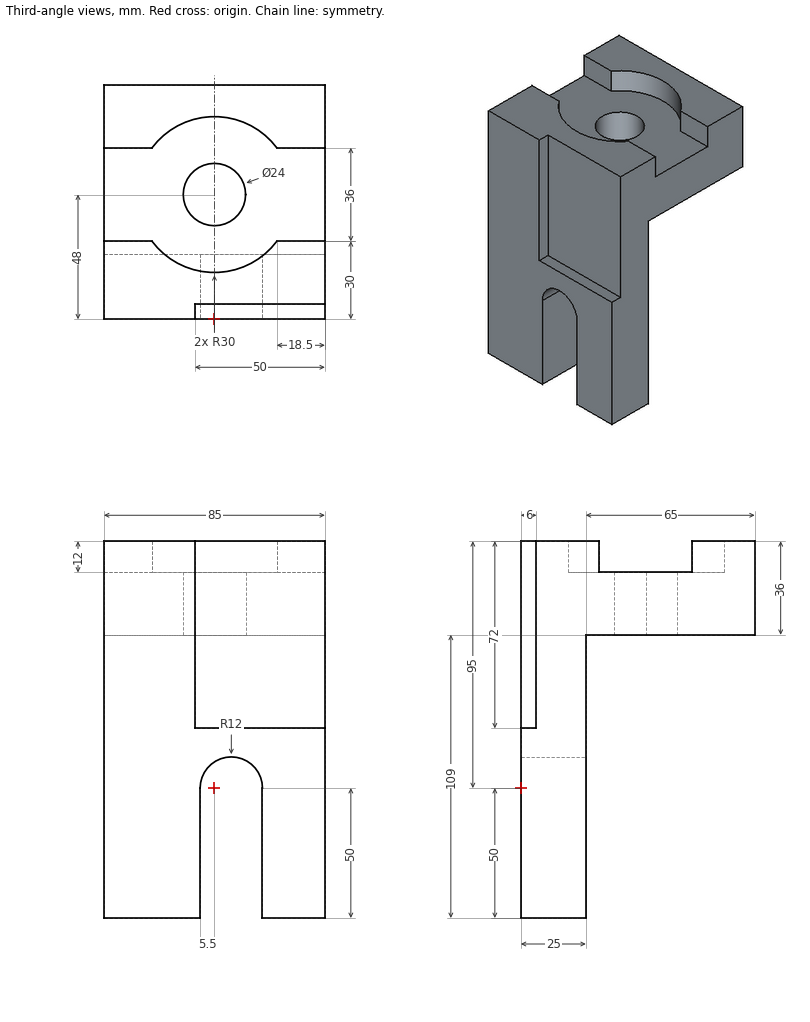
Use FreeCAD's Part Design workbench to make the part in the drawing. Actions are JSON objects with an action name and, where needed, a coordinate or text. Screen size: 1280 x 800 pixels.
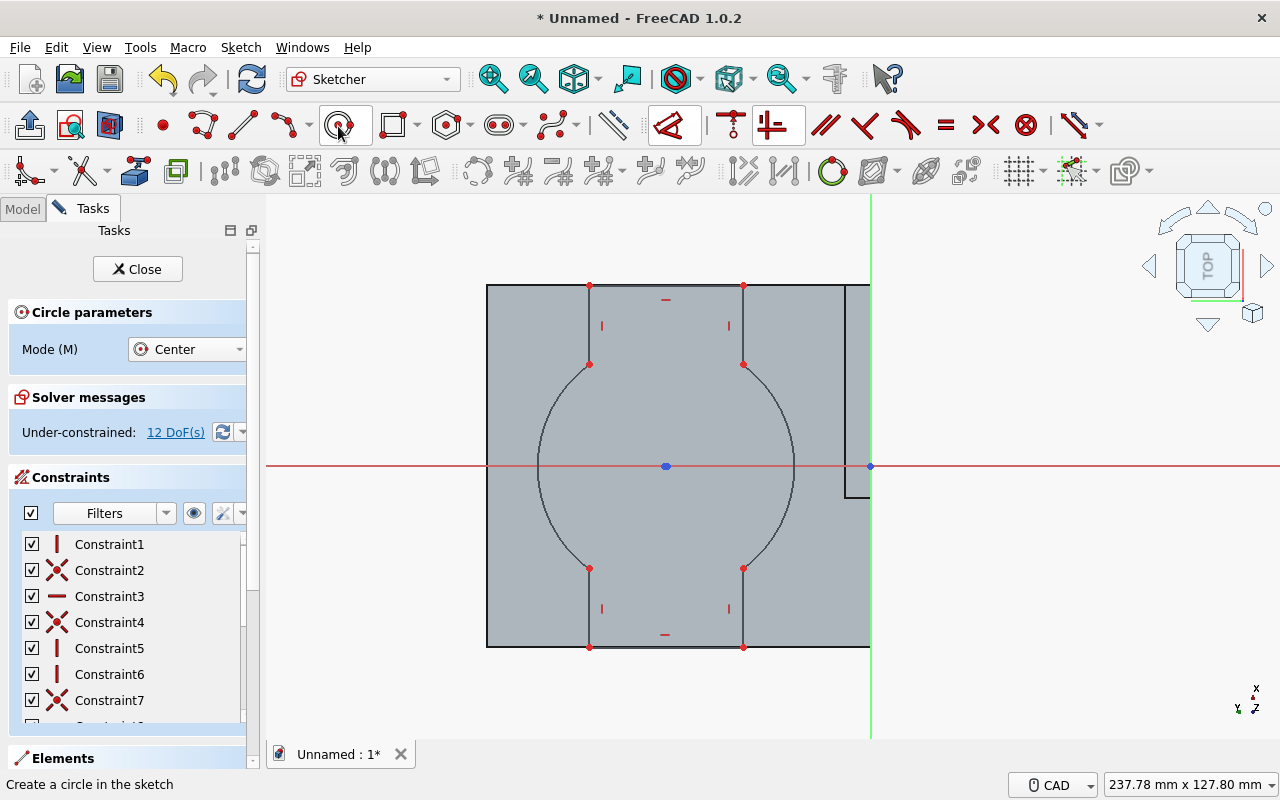
{"action": "left_click", "coordinate": [666, 466]}
{"action": "left_click", "coordinate": [702, 430]}
{"action": "key", "text": "Escape"}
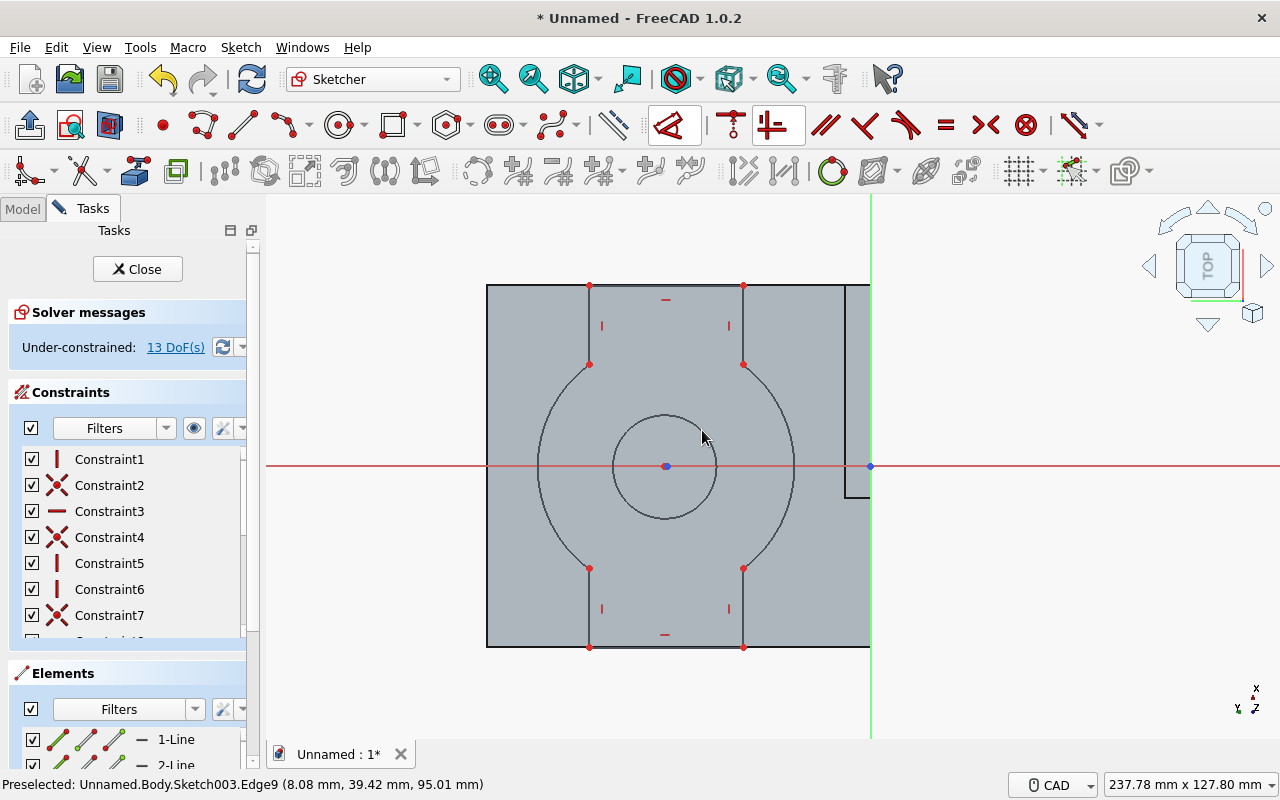
{"action": "left_click", "coordinate": [701, 430]}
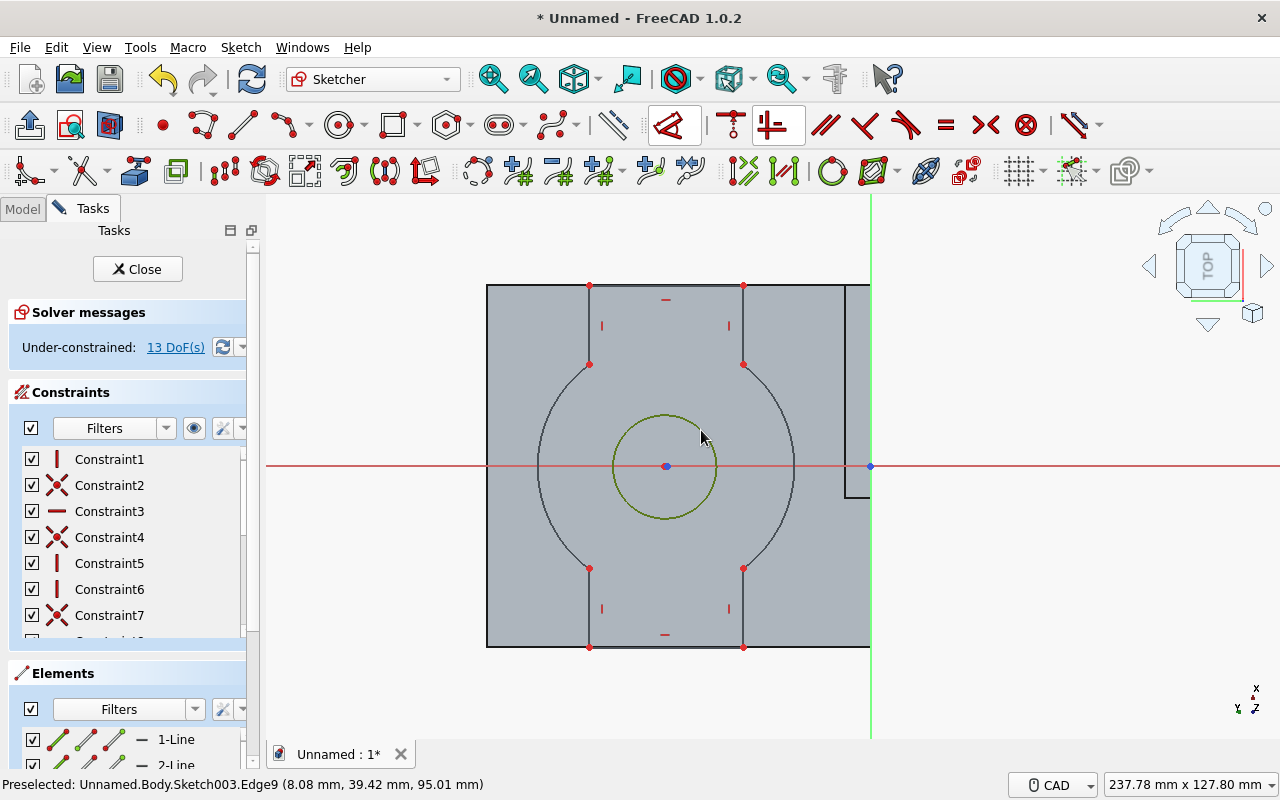
{"action": "left_click", "coordinate": [786, 513]}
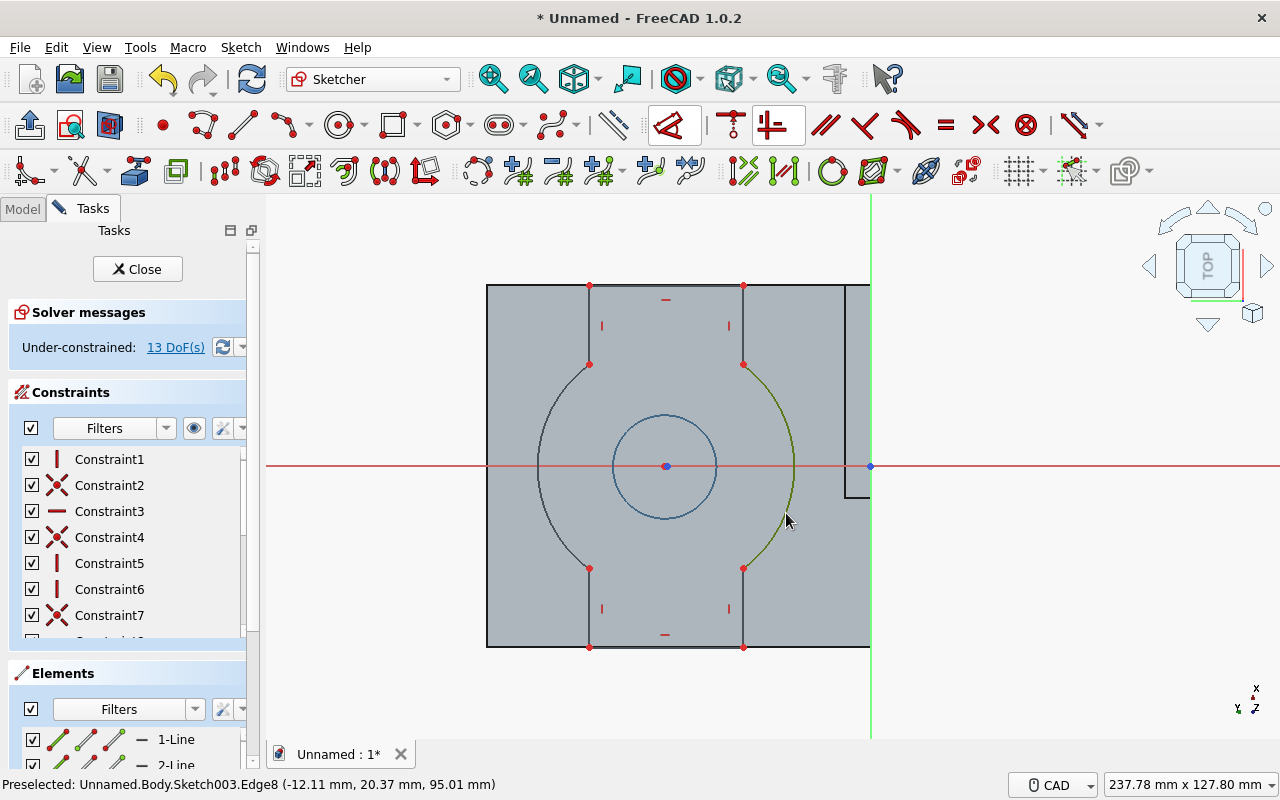
{"action": "left_click", "coordinate": [732, 126]}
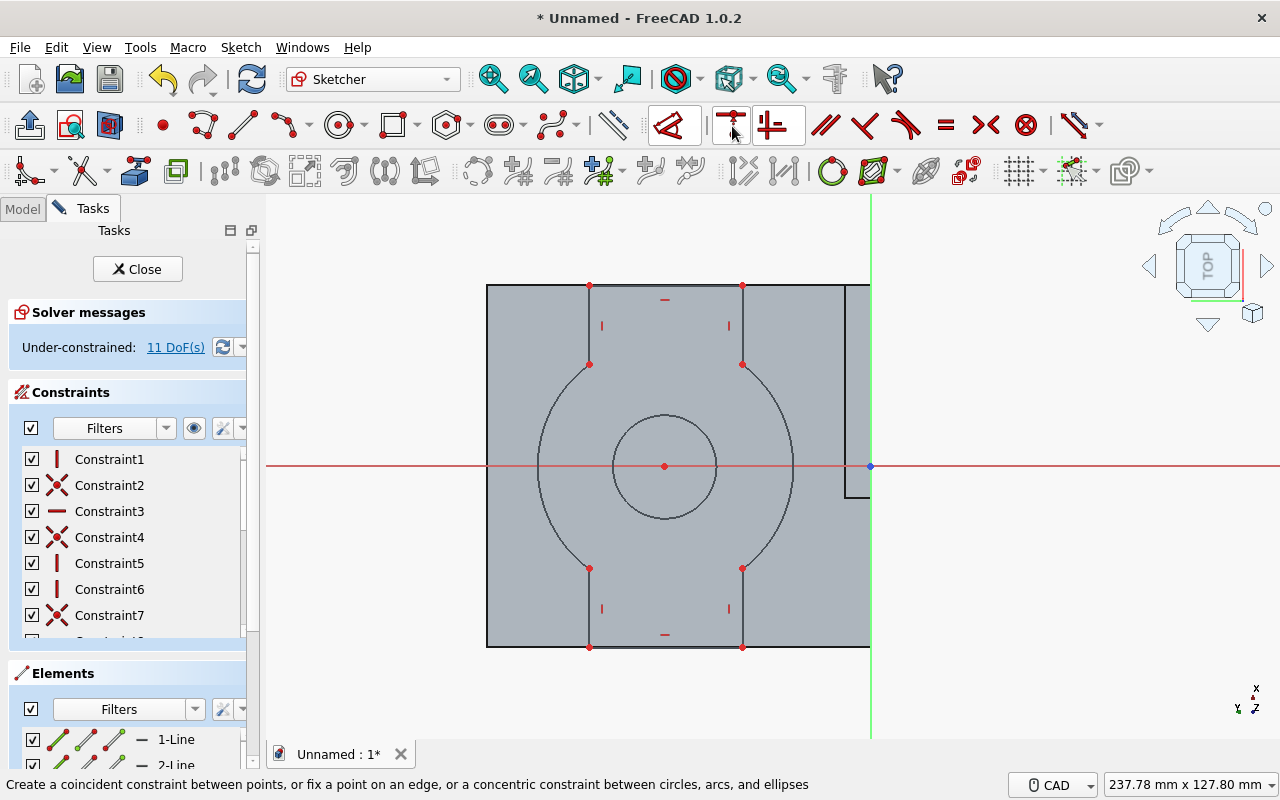
{"action": "left_click", "coordinate": [546, 421]}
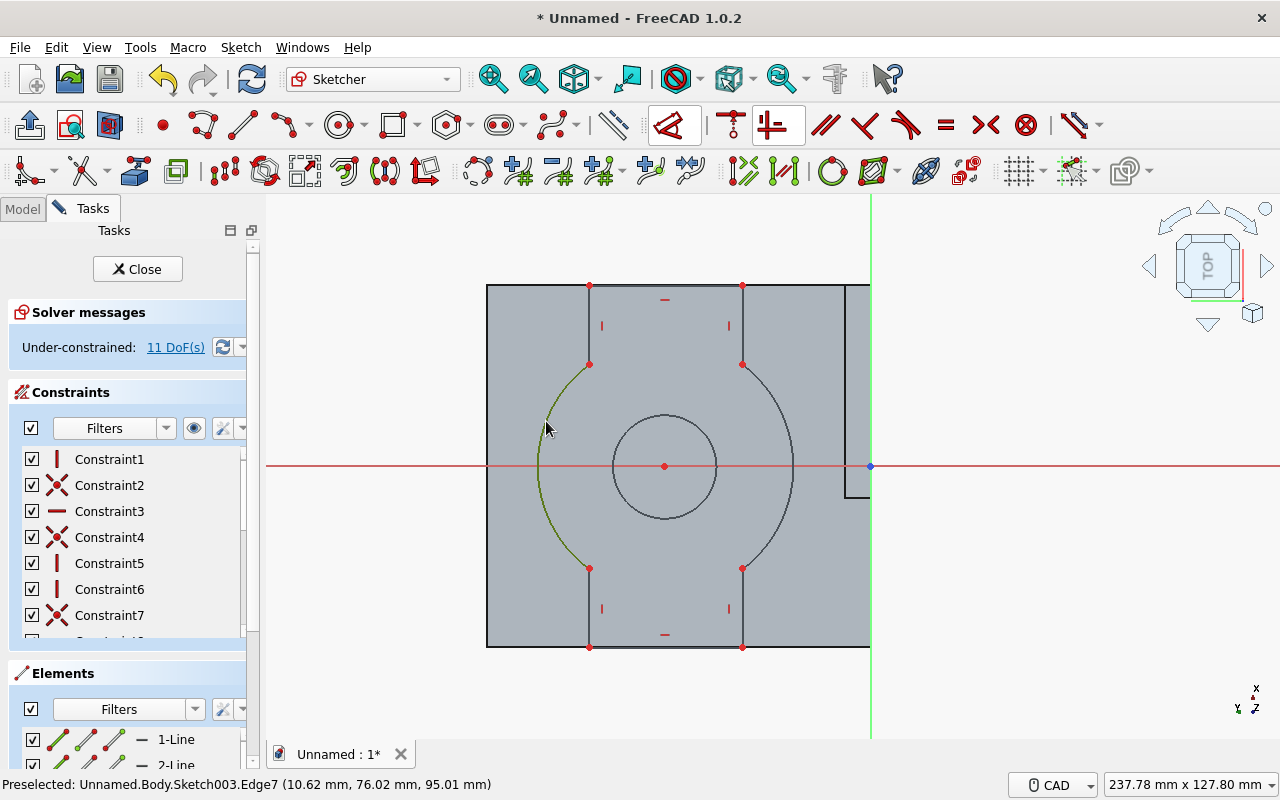
{"action": "left_click", "coordinate": [785, 513]}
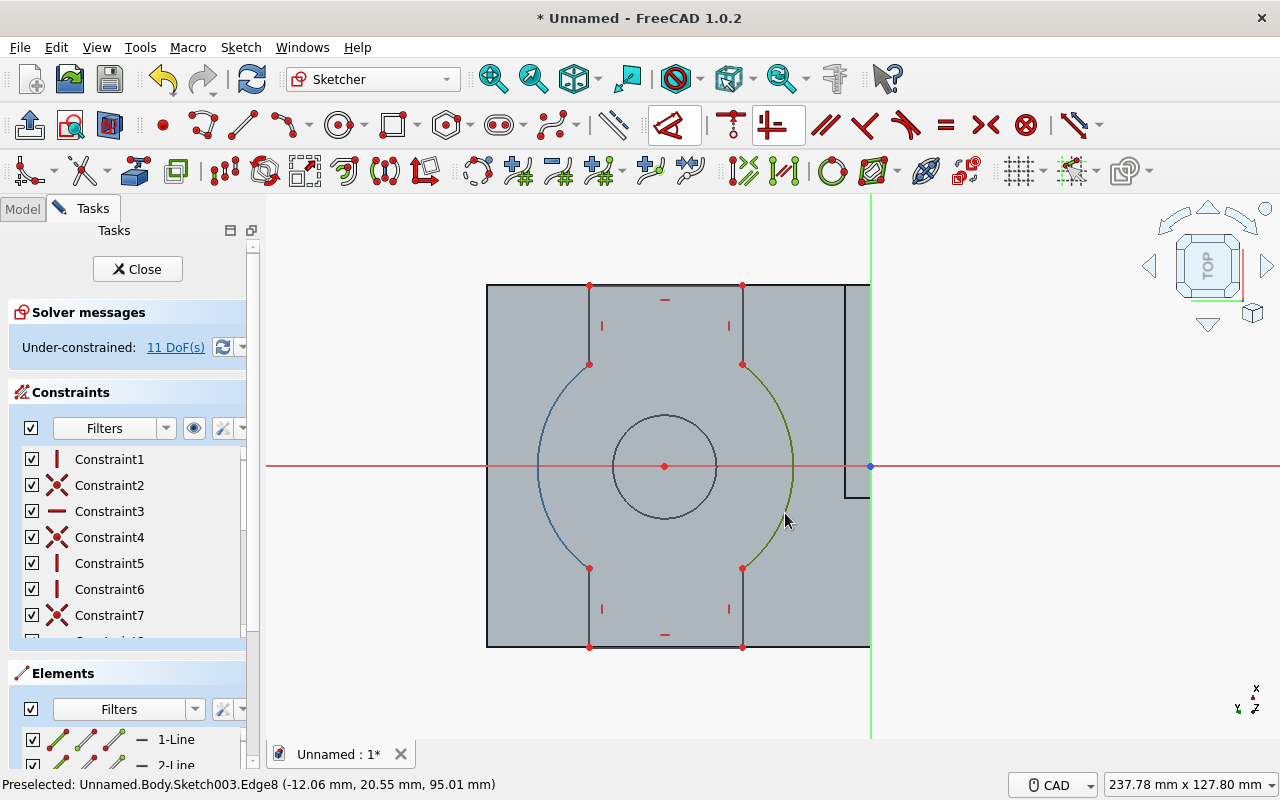
{"action": "left_click", "coordinate": [946, 126]}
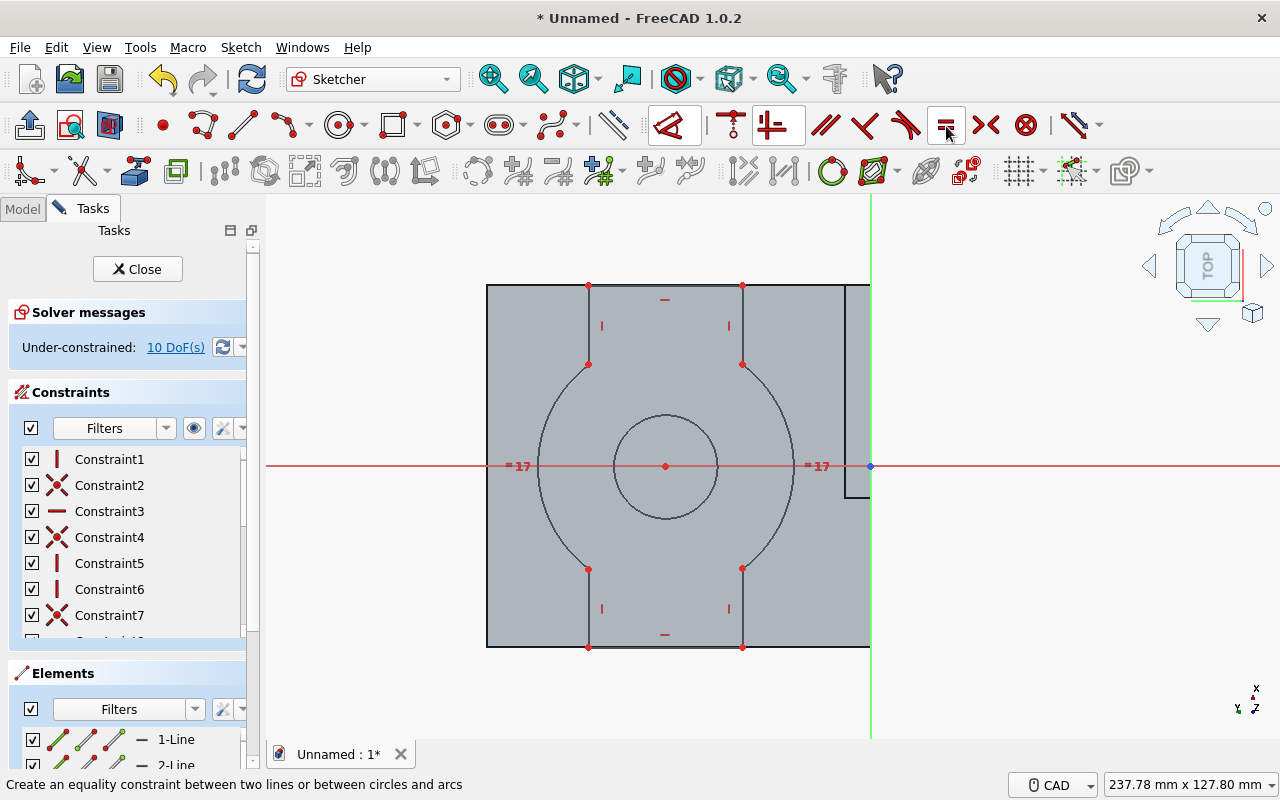
{"action": "left_click", "coordinate": [666, 467]}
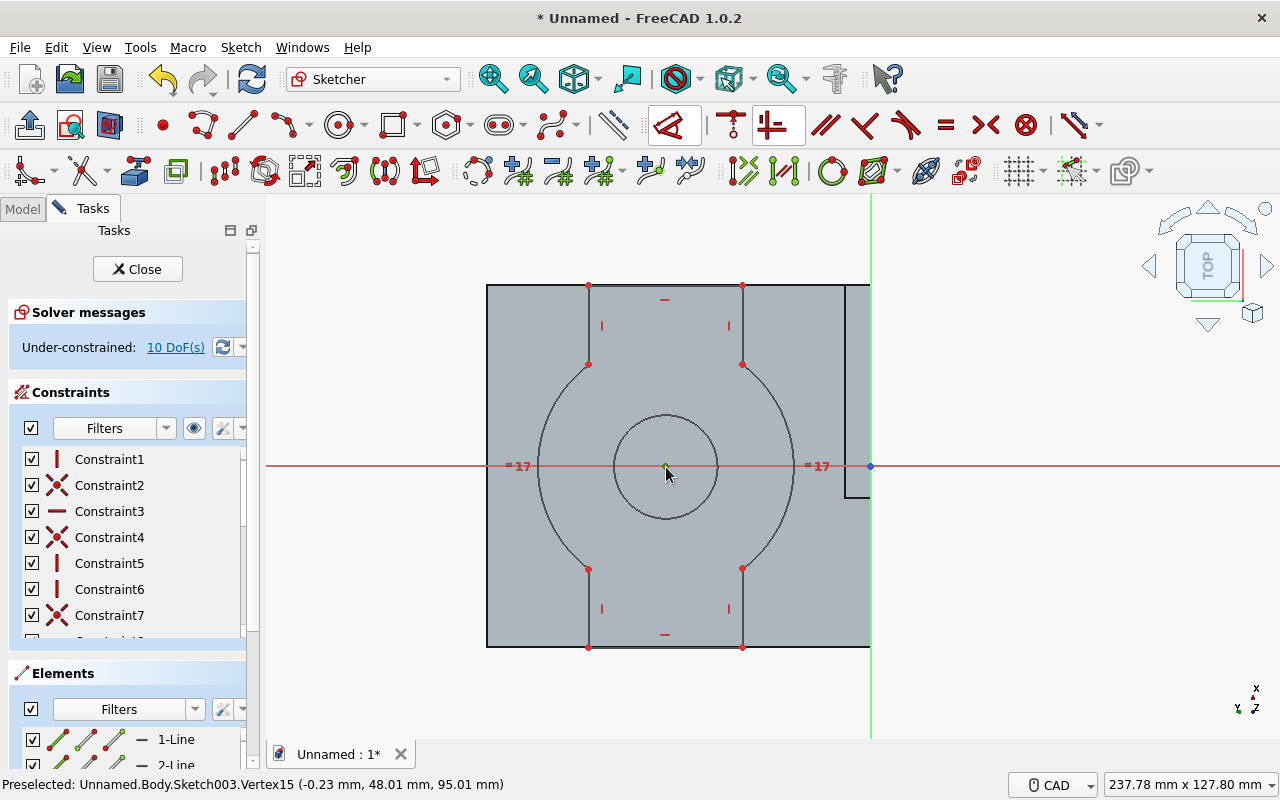
{"action": "left_click", "coordinate": [353, 466]}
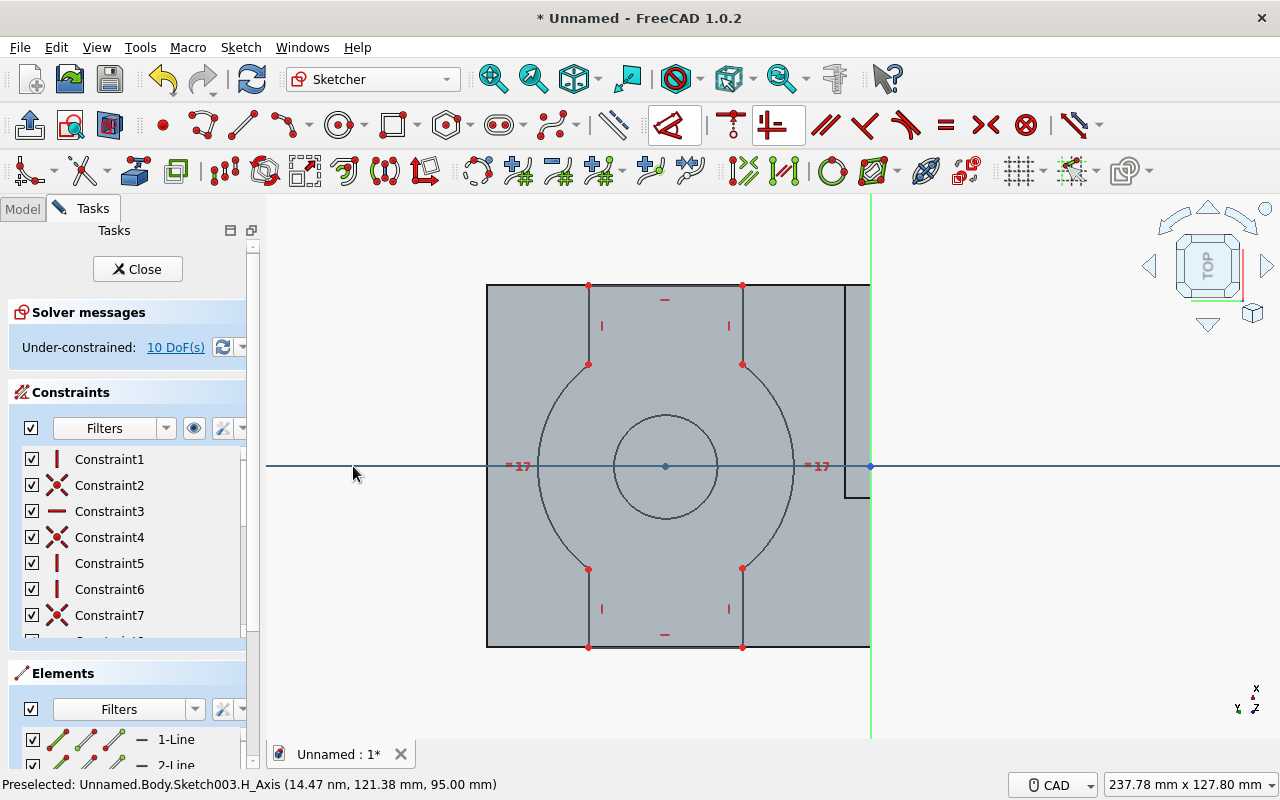
{"action": "left_click", "coordinate": [732, 126]}